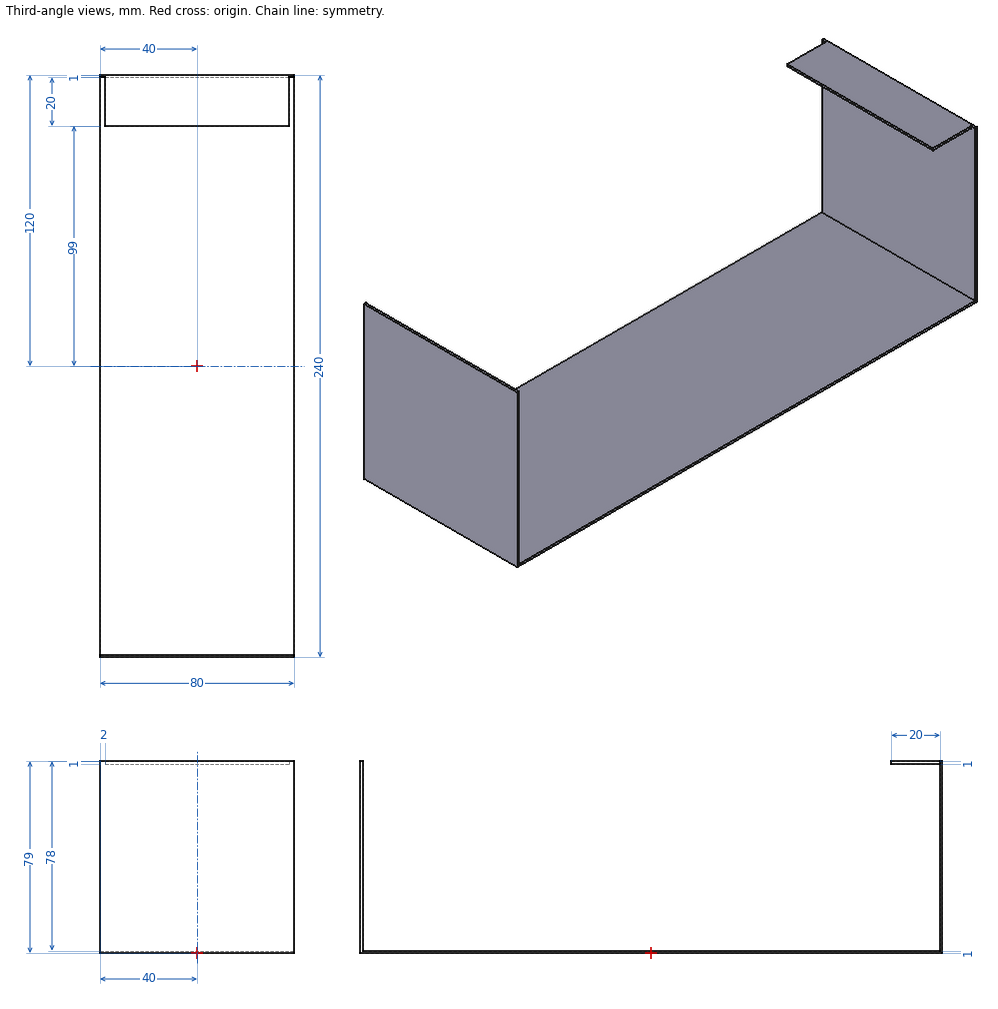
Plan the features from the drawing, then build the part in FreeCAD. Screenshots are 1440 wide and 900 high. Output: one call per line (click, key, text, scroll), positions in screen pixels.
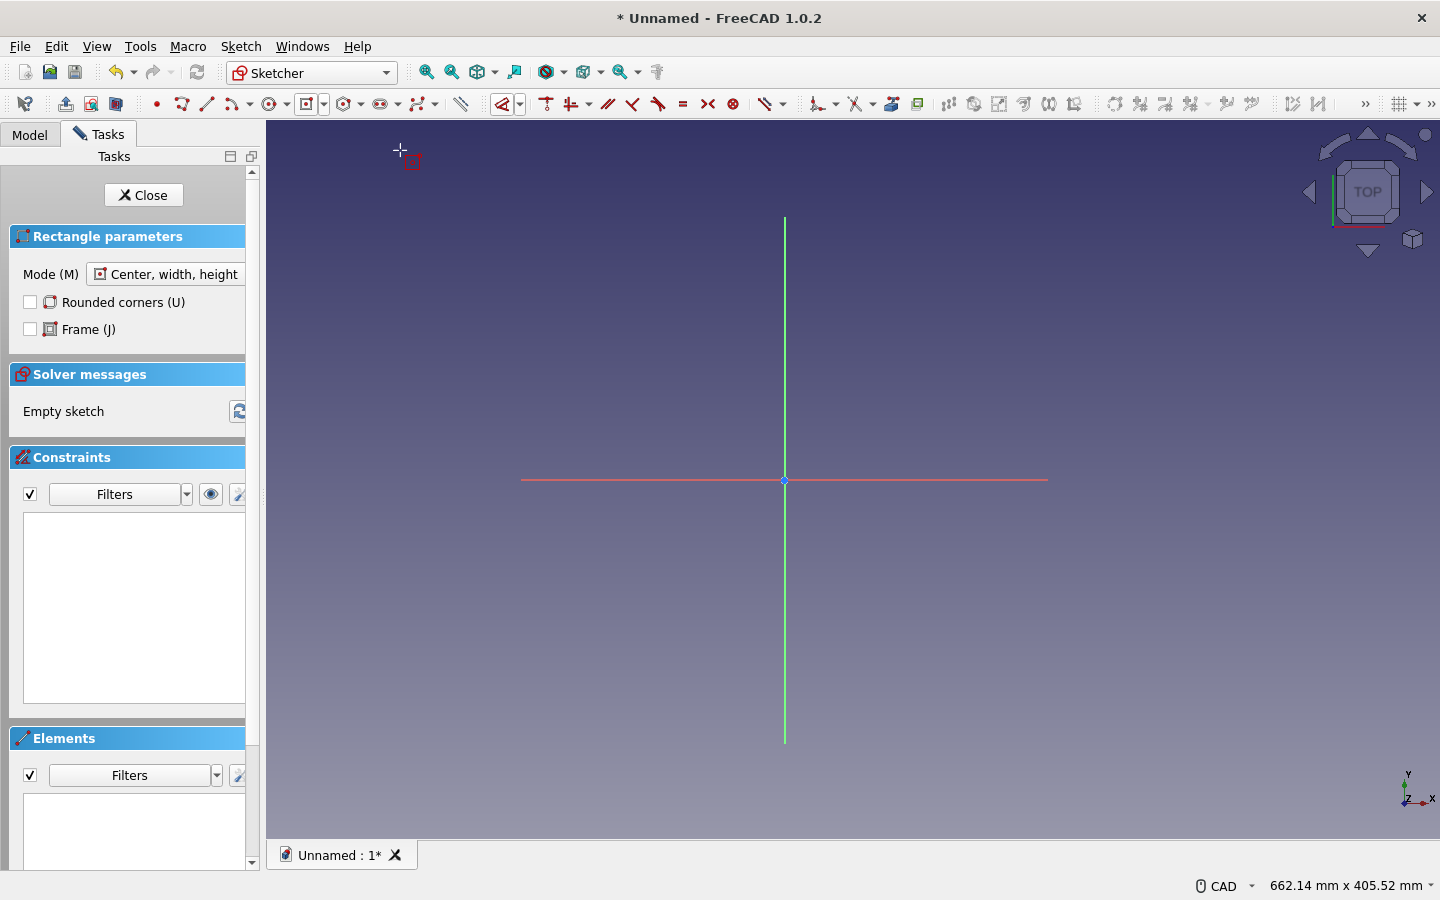
click(785, 480)
click(856, 267)
key(Escape)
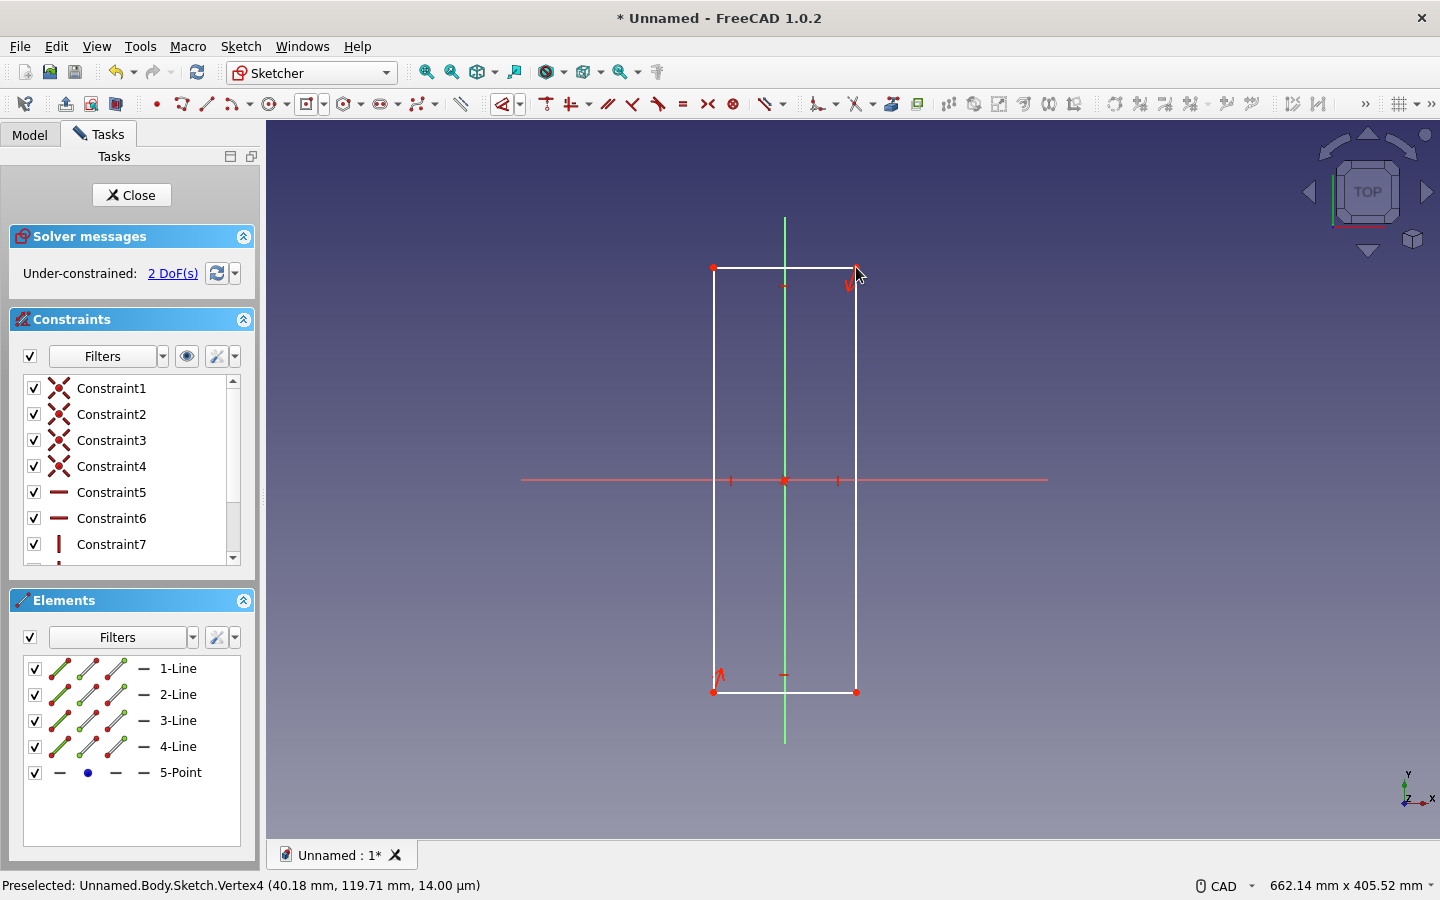
click(502, 104)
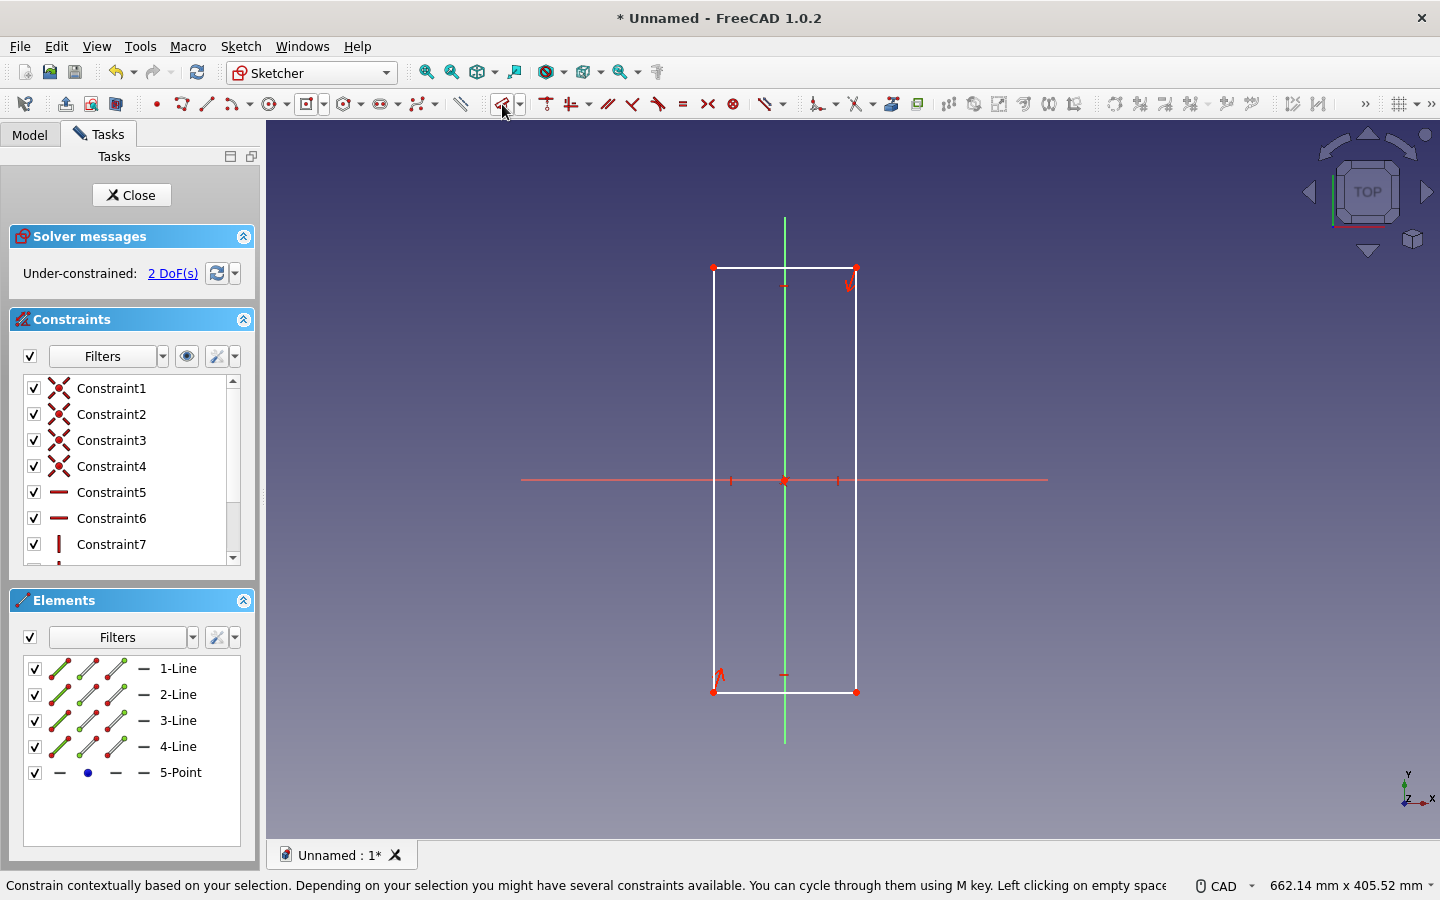
click(756, 693)
click(752, 727)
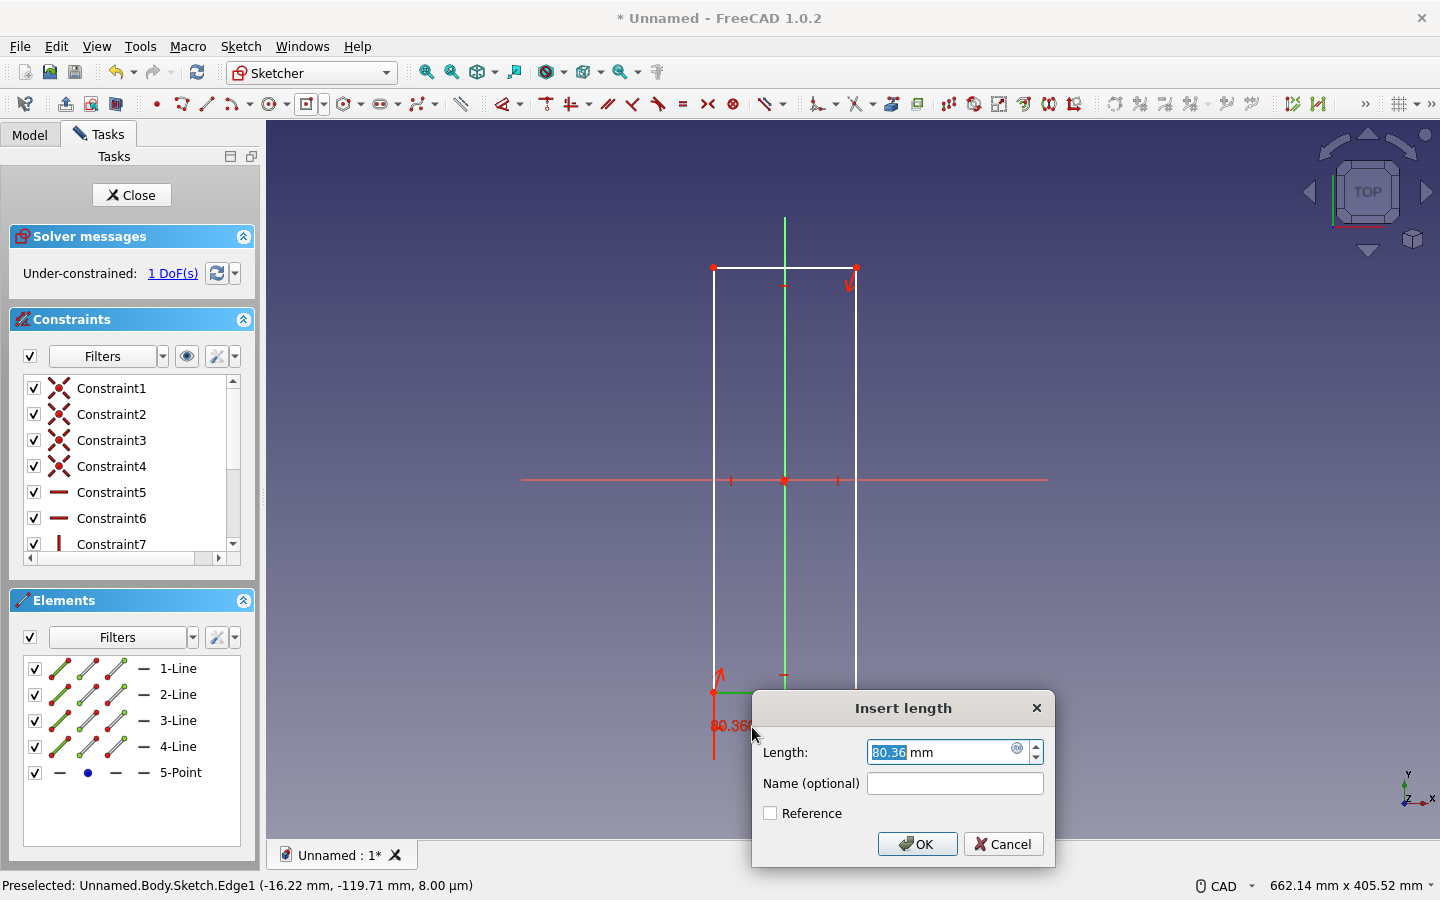
text(80)
key(Return)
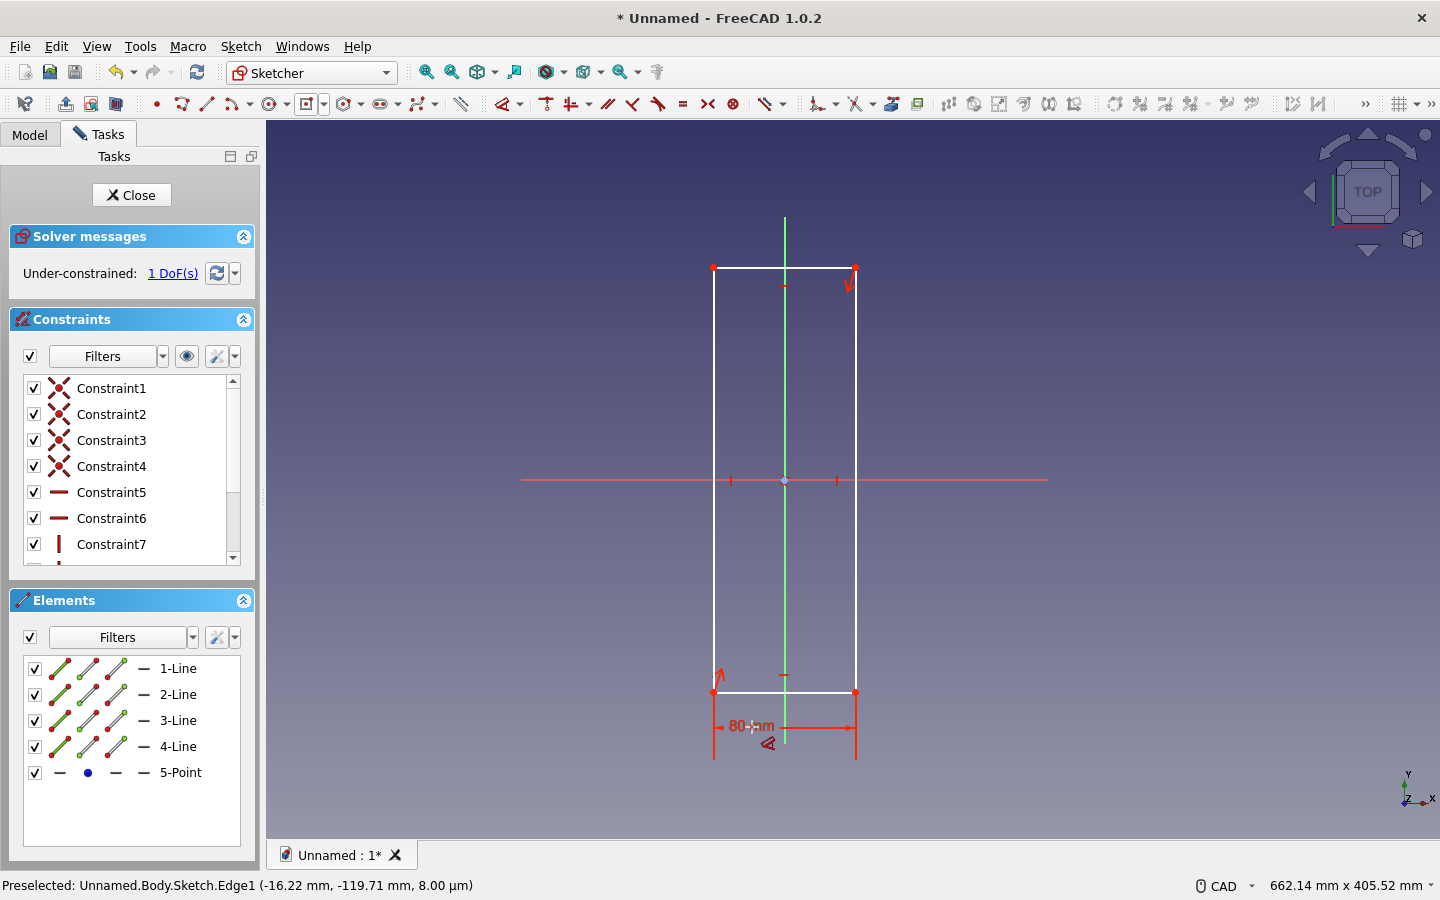
click(856, 565)
click(890, 383)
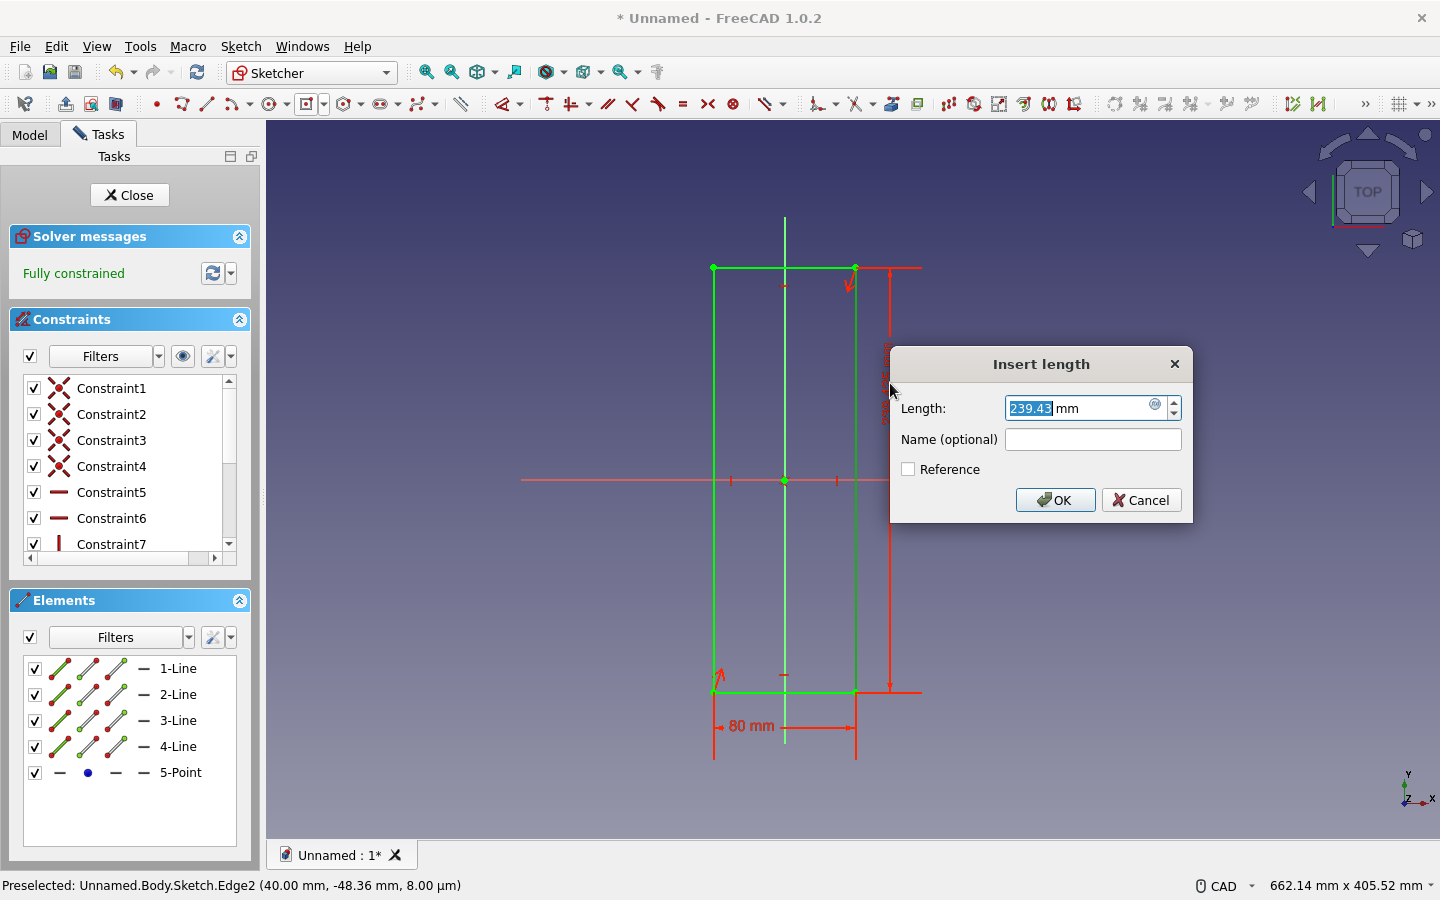
text(240)
key(Return)
key(Escape)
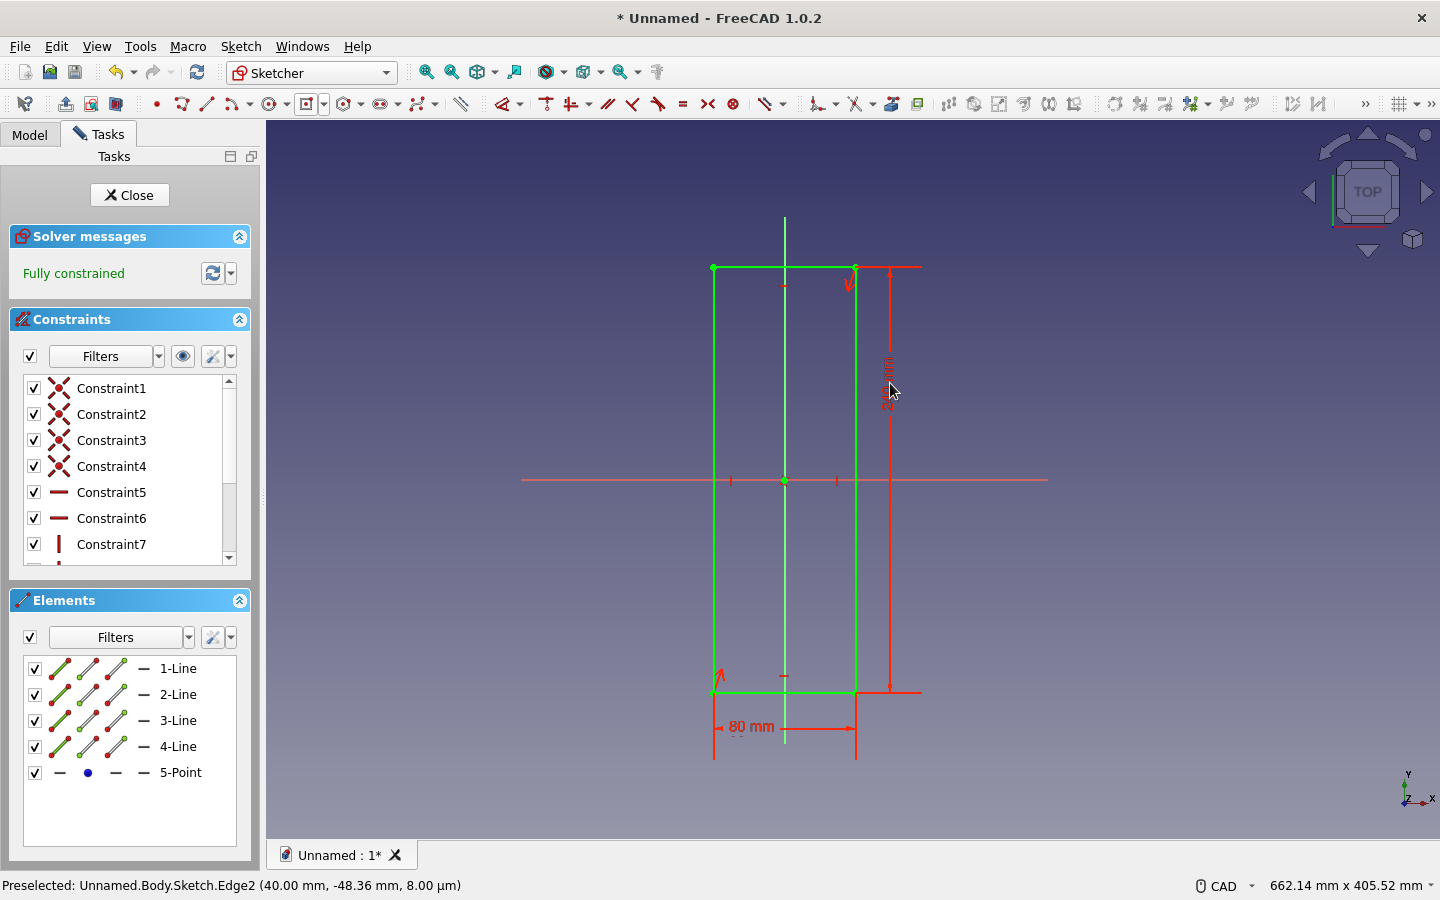
click(130, 195)